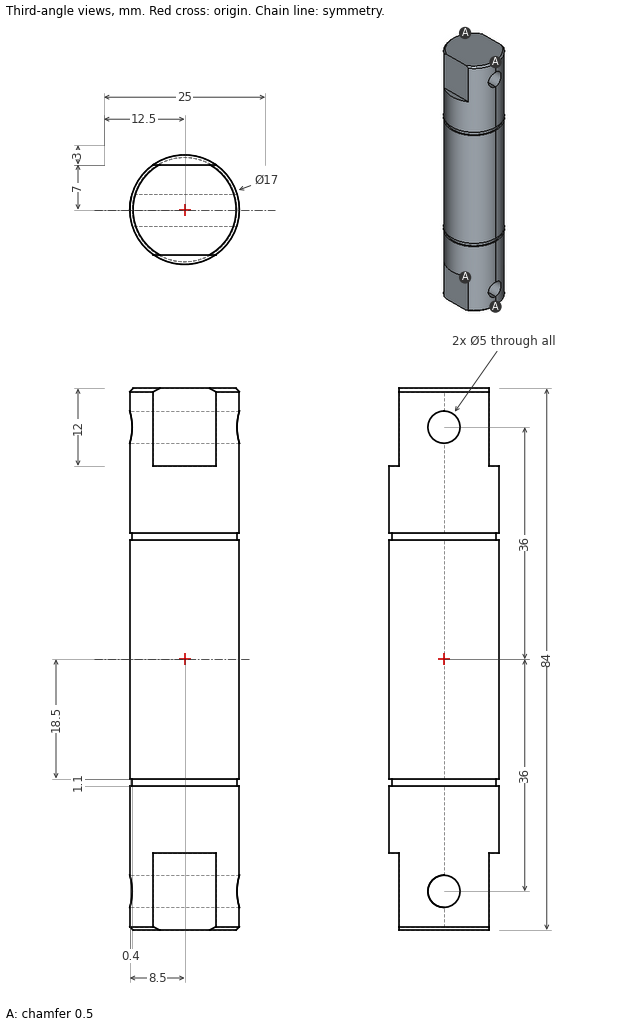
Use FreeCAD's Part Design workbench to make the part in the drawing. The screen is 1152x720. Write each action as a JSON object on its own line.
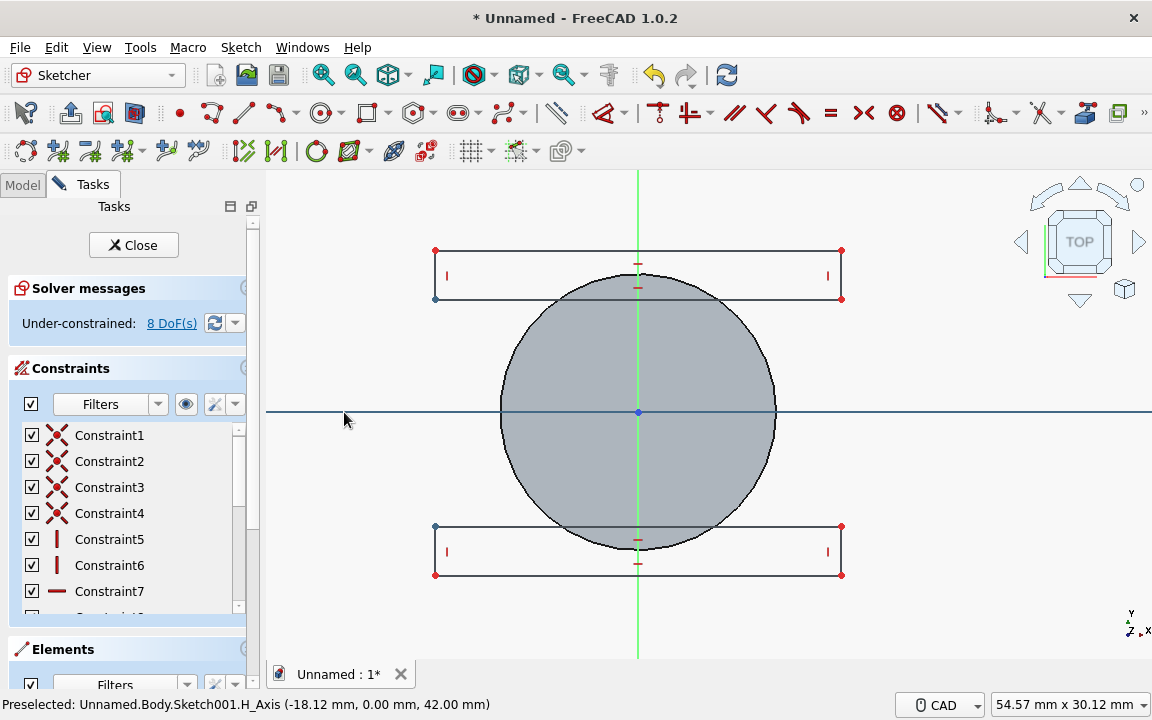
{"action": "left_click", "coordinate": [864, 114]}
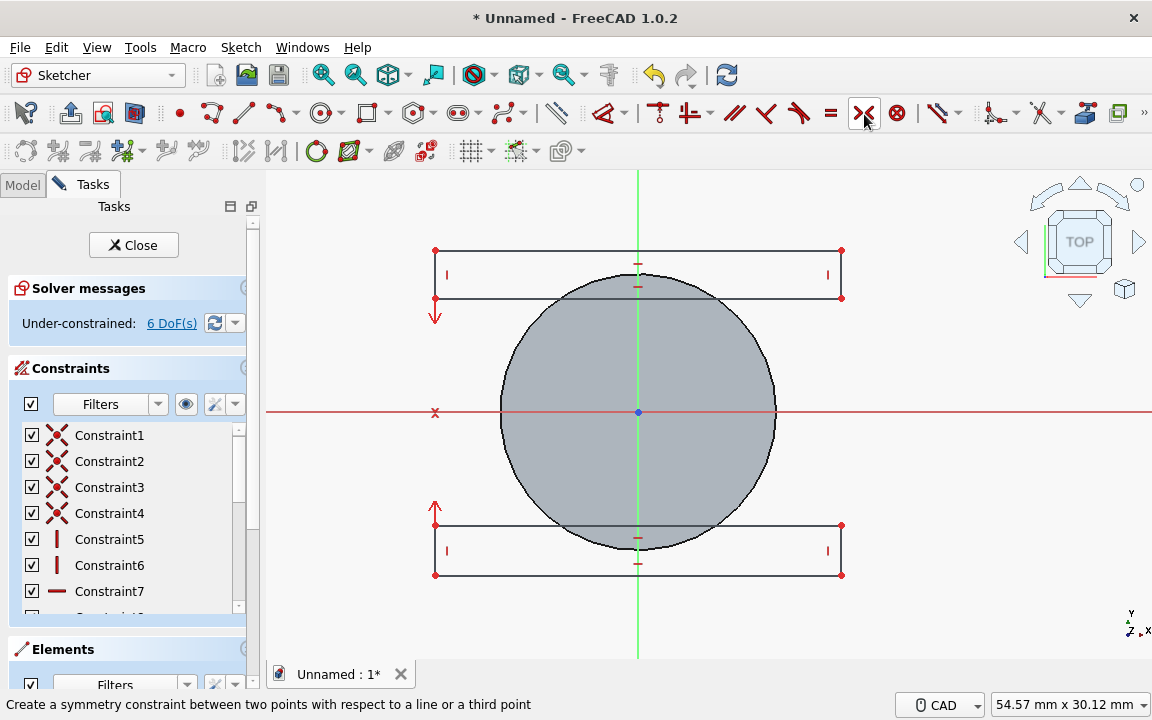
{"action": "left_click", "coordinate": [841, 251]}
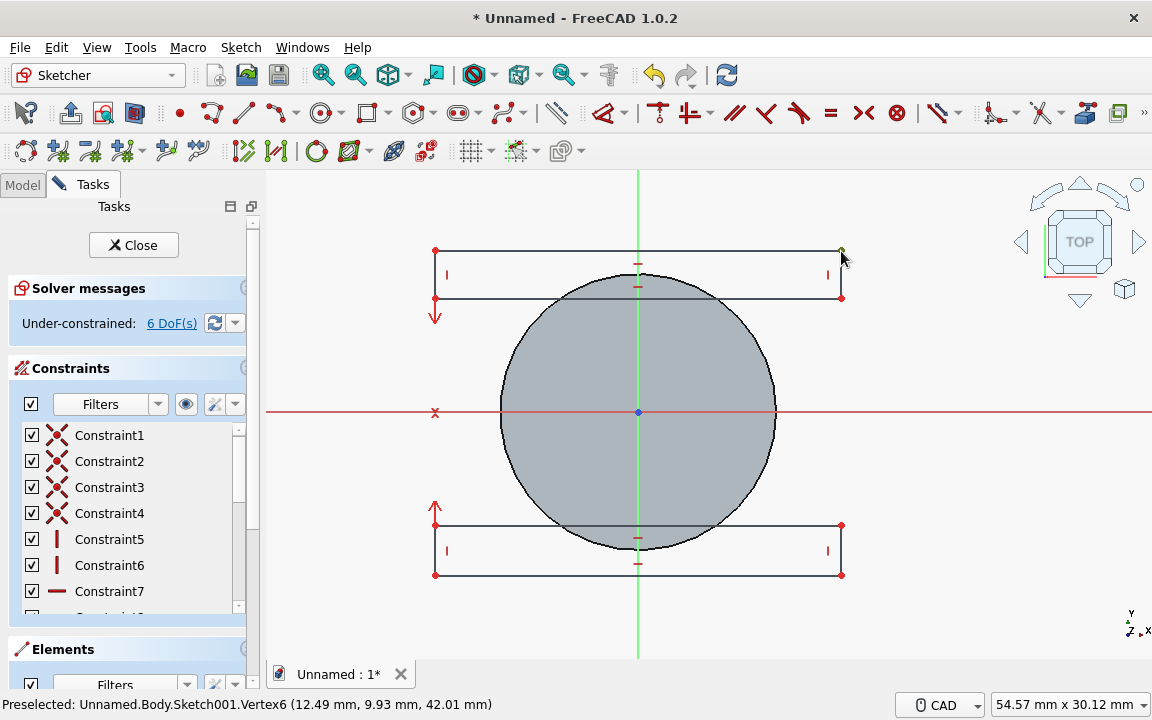
{"action": "left_click", "coordinate": [841, 576]}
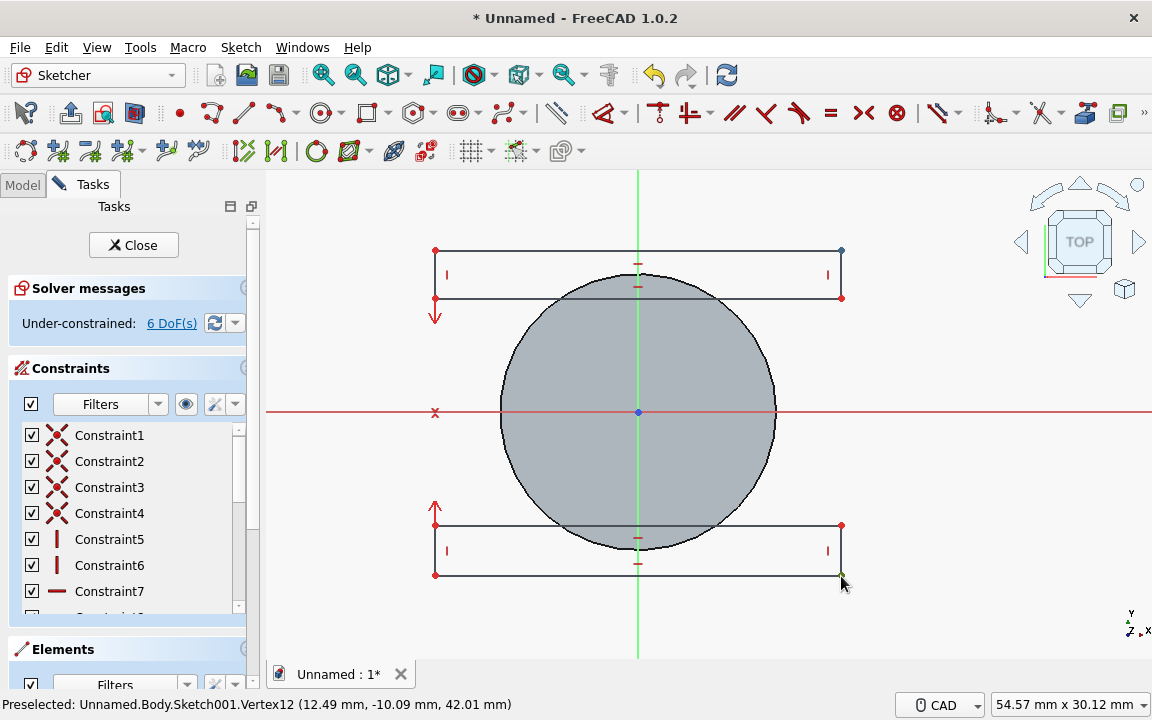
{"action": "left_click", "coordinate": [344, 412]}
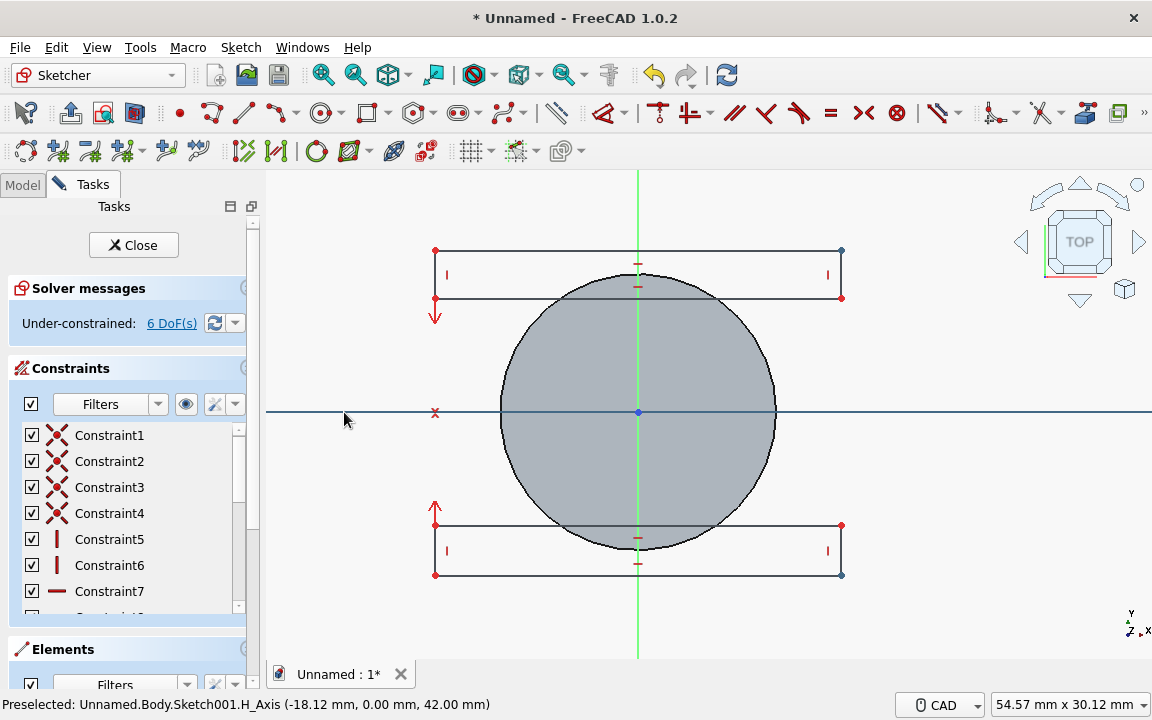
{"action": "left_click", "coordinate": [864, 114]}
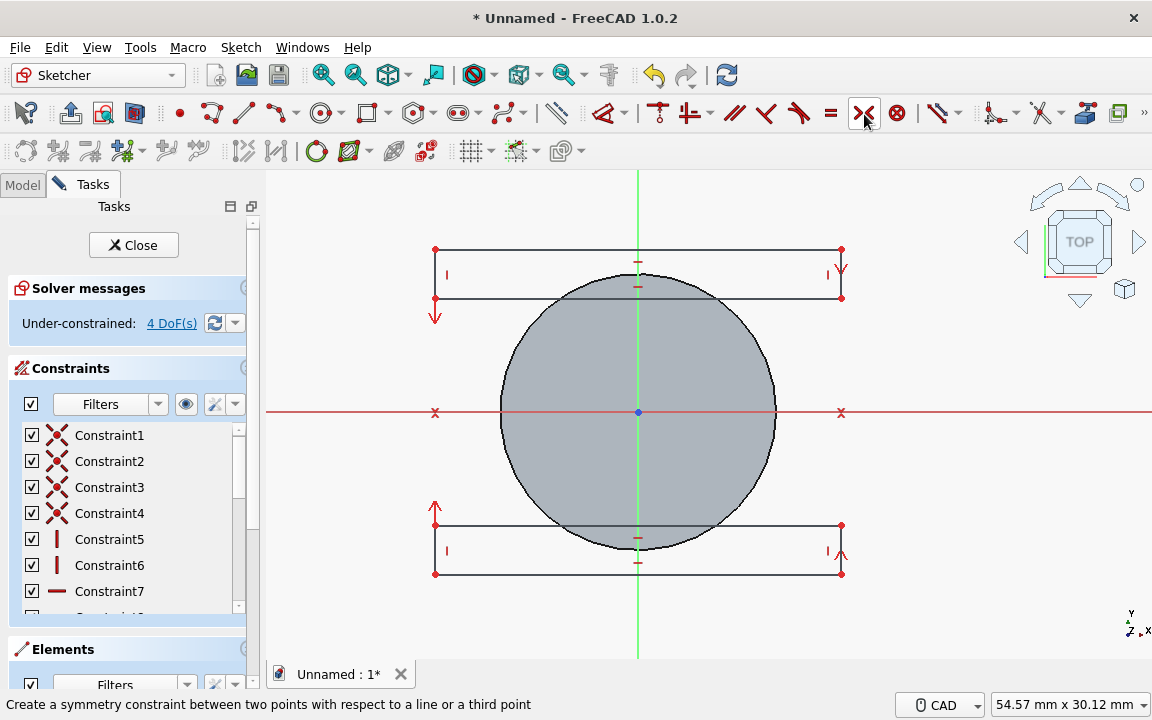
{"action": "left_click", "coordinate": [604, 114]}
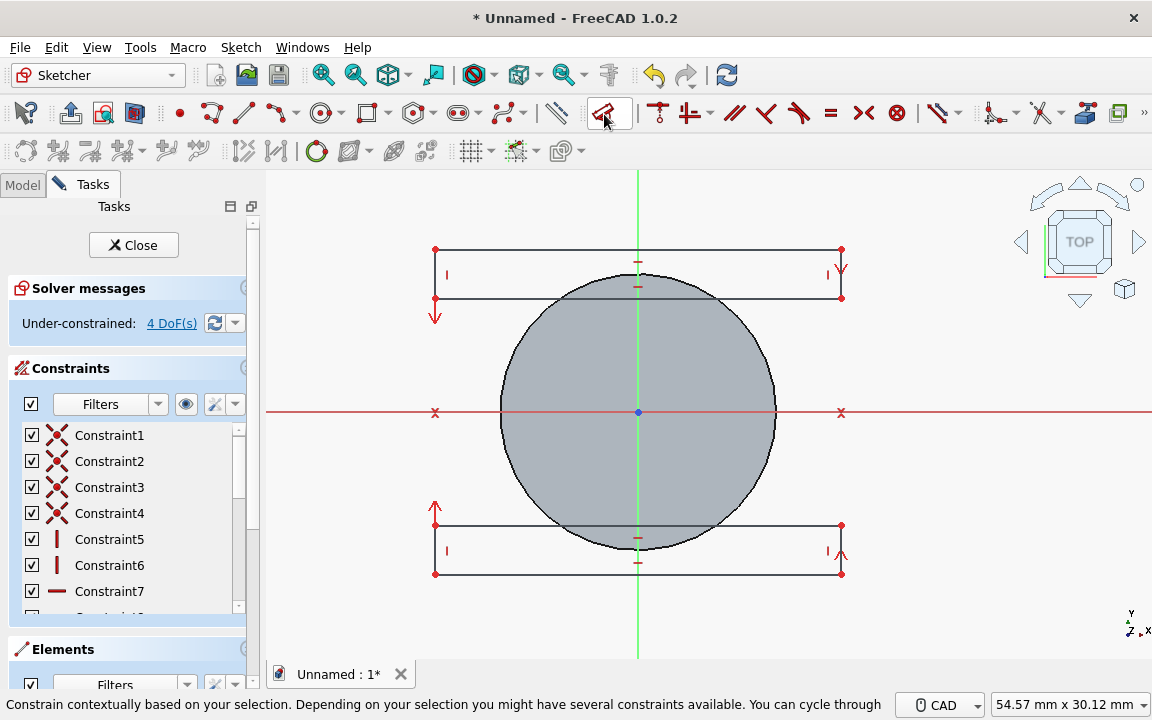
{"action": "left_click", "coordinate": [435, 264]}
{"action": "left_click", "coordinate": [401, 274]}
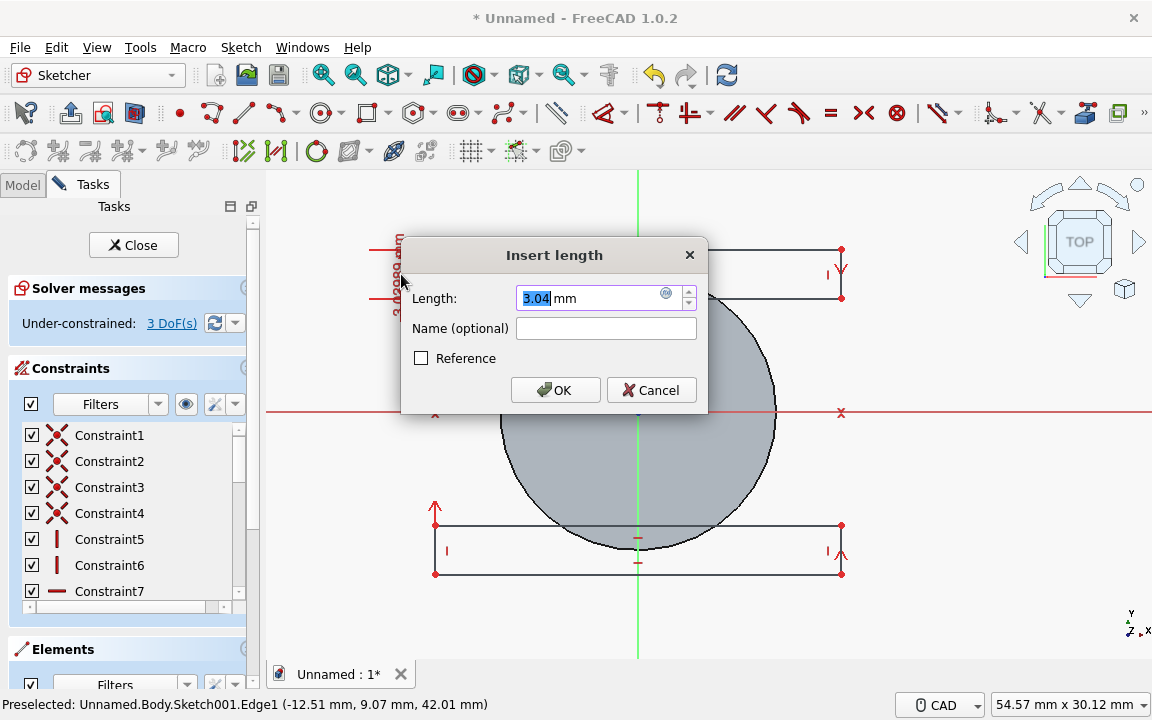
{"action": "type", "text": "3"}
{"action": "key", "text": "Return"}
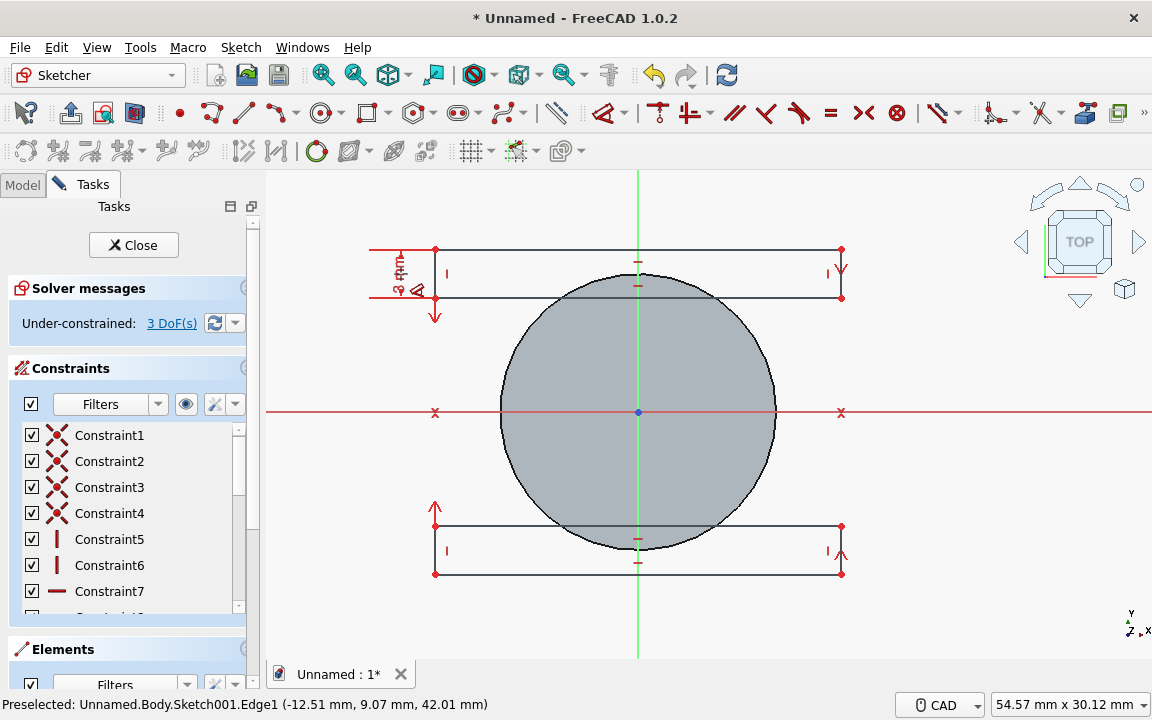
{"action": "left_click", "coordinate": [557, 298]}
{"action": "left_click", "coordinate": [545, 264]}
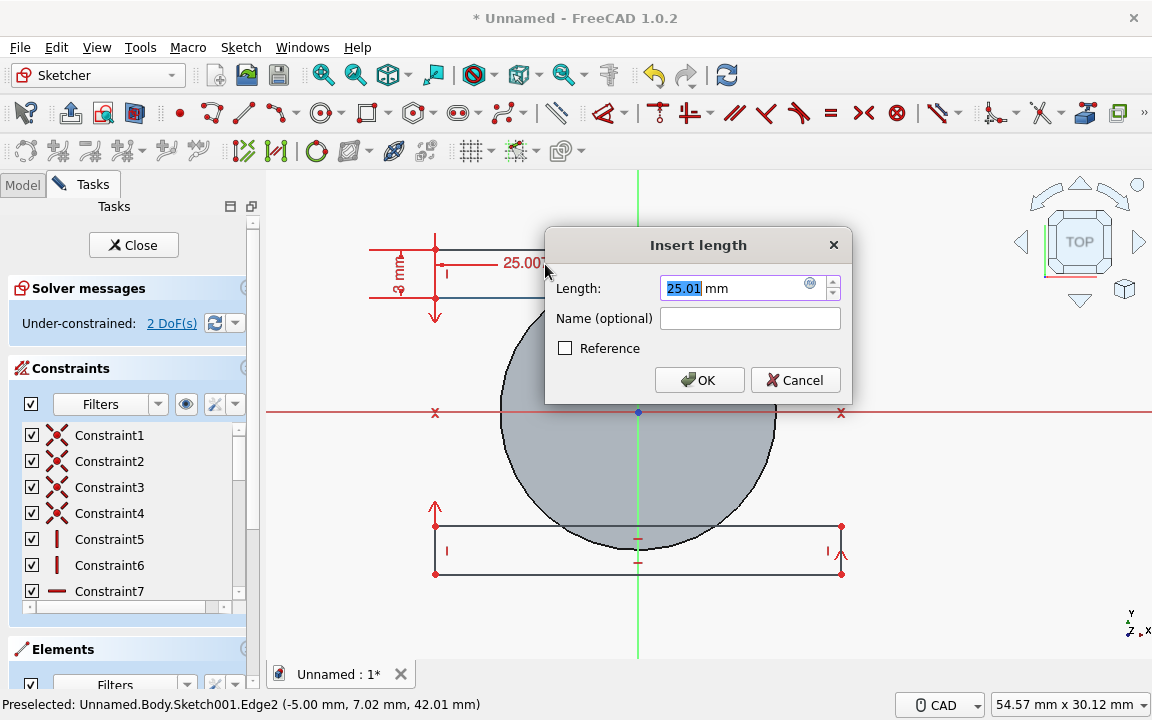
{"action": "type", "text": "25"}
{"action": "key", "text": "Return"}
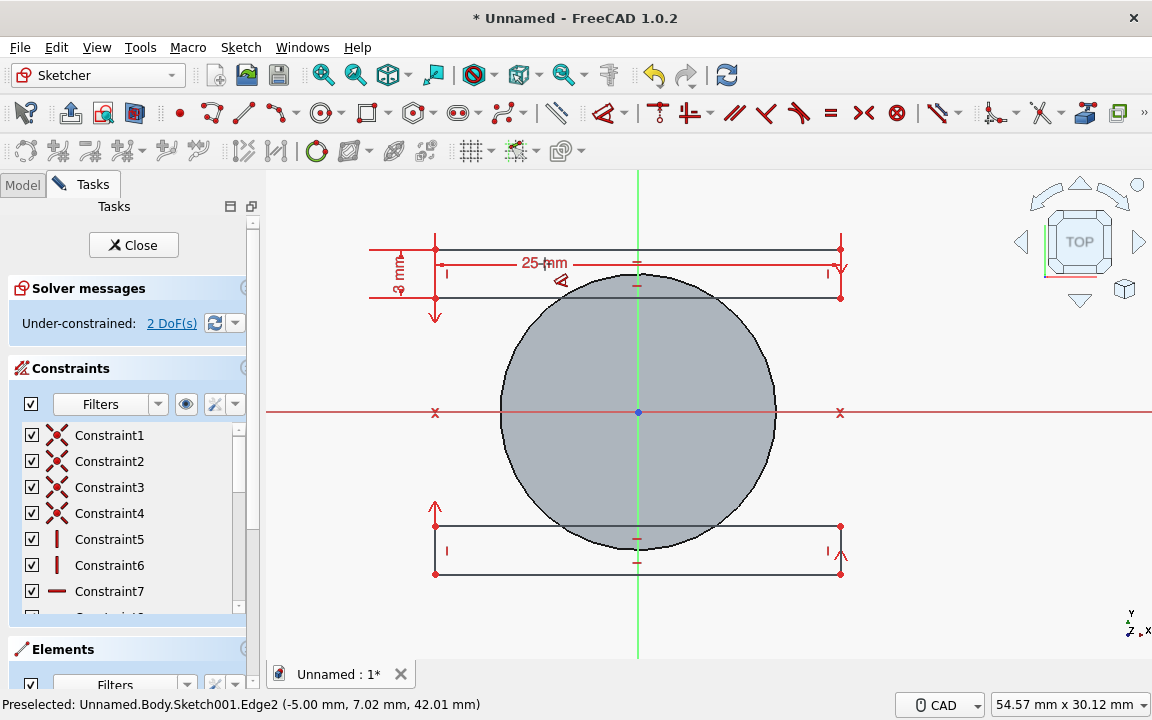
{"action": "left_click", "coordinate": [435, 298]}
{"action": "left_click", "coordinate": [401, 355]}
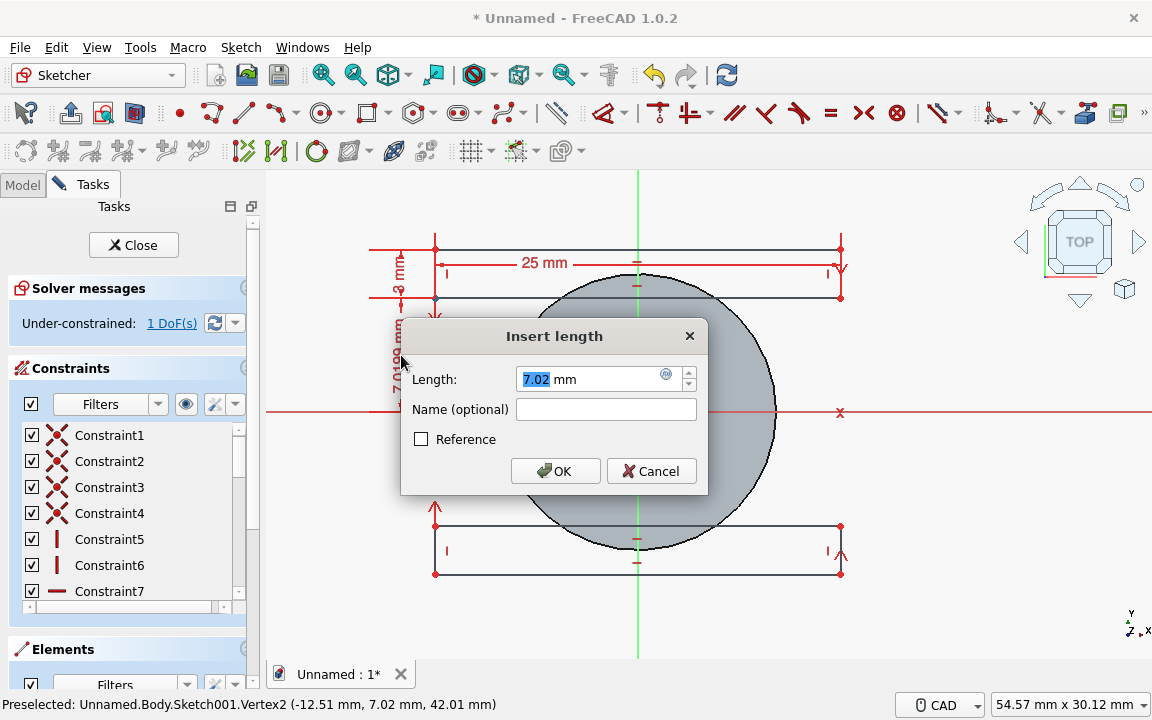
{"action": "type", "text": "7"}
{"action": "key", "text": "Return"}